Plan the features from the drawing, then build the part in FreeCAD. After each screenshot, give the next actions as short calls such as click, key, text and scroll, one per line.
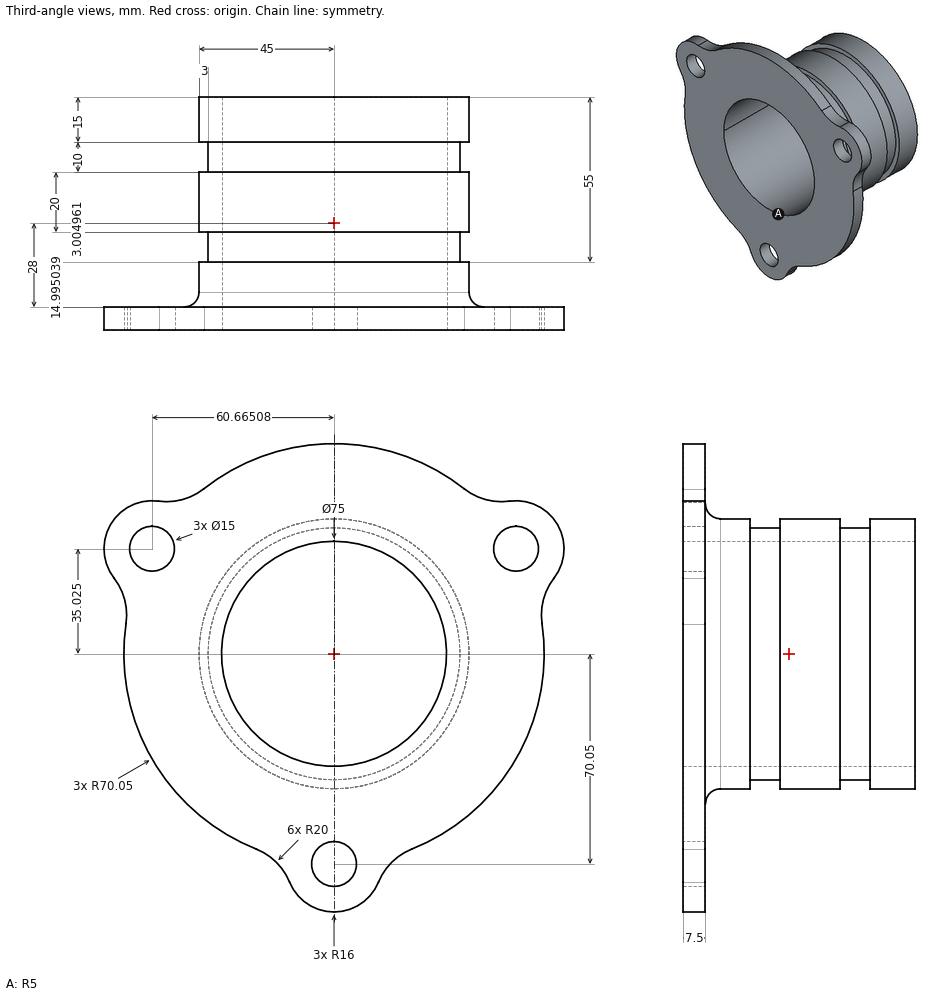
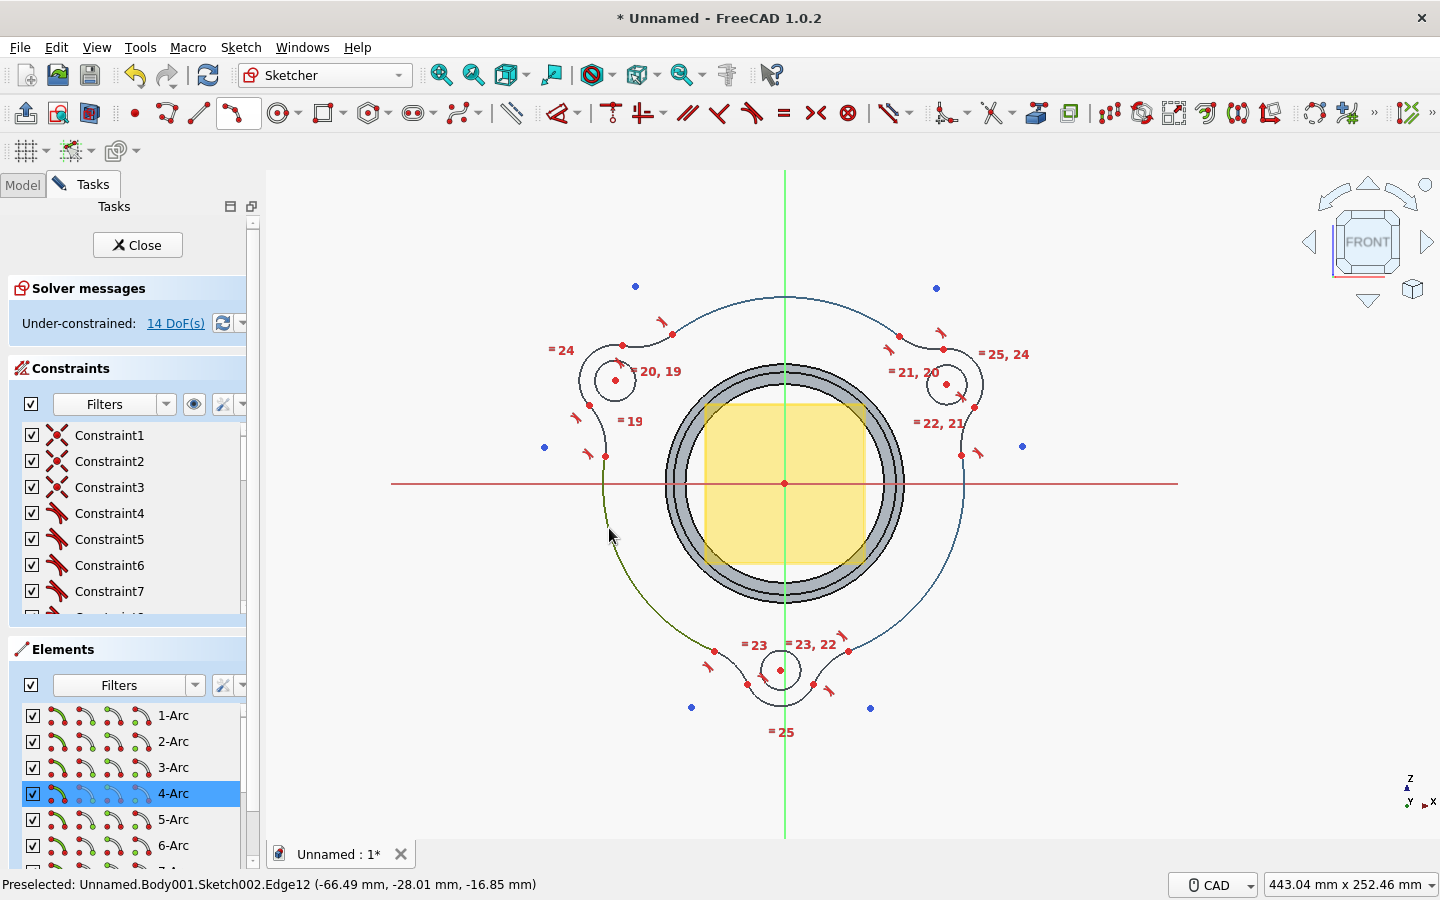
click(784, 114)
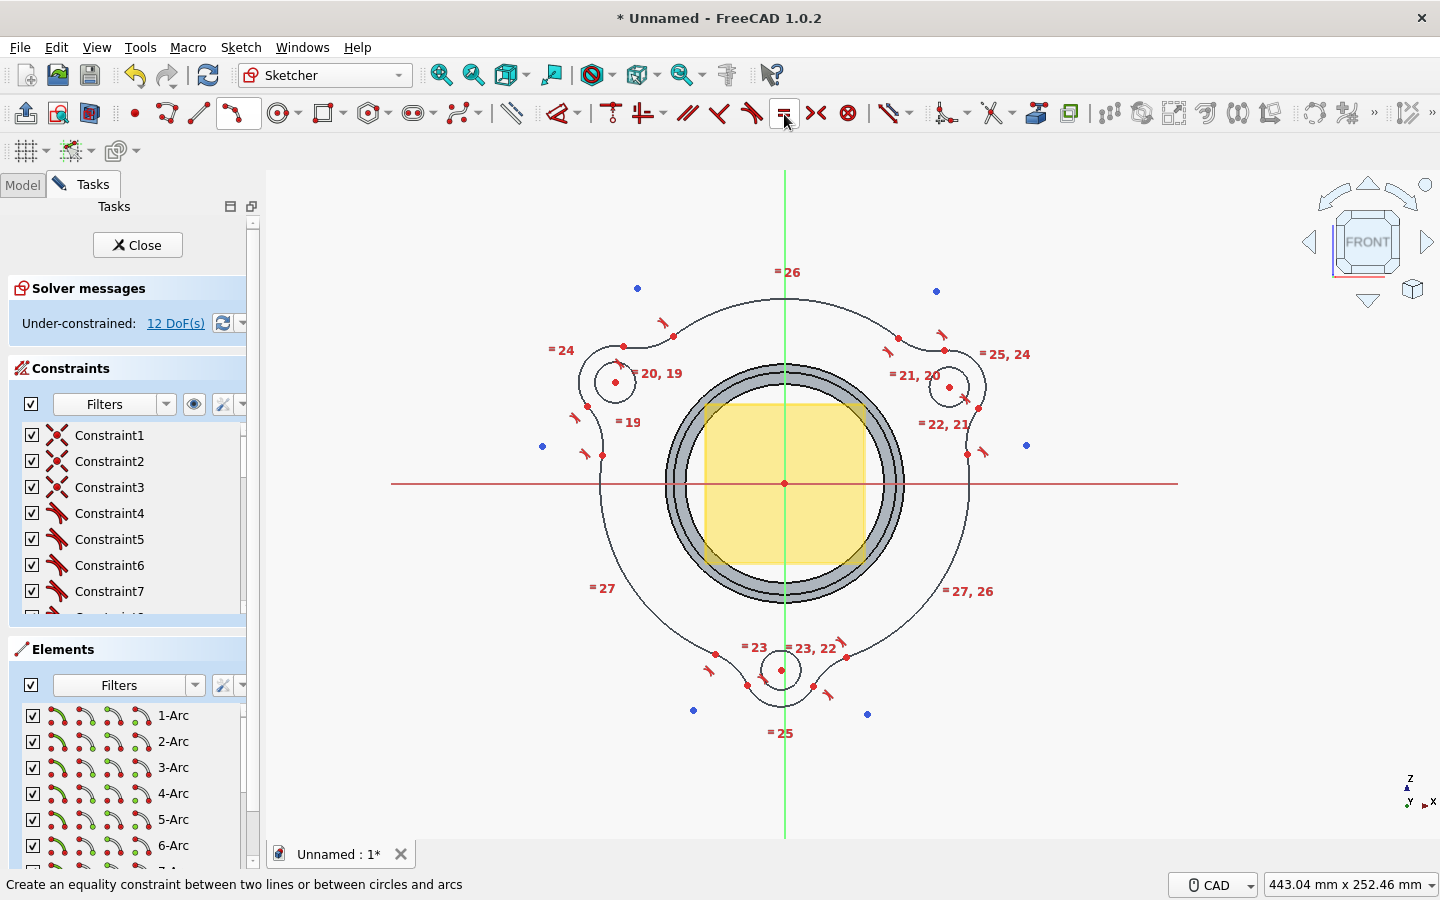
click(601, 368)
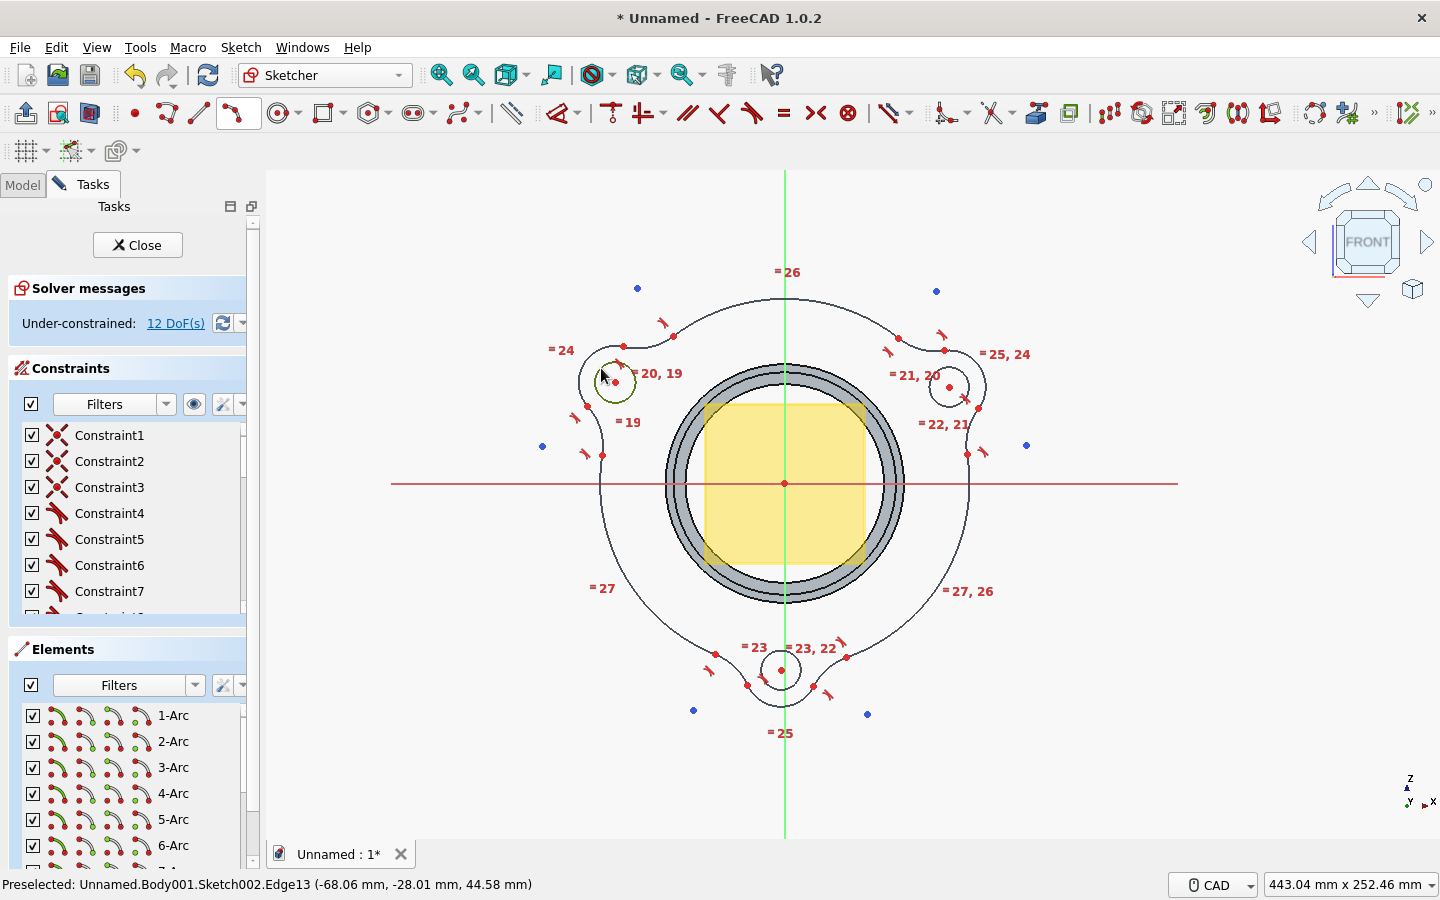
click(963, 373)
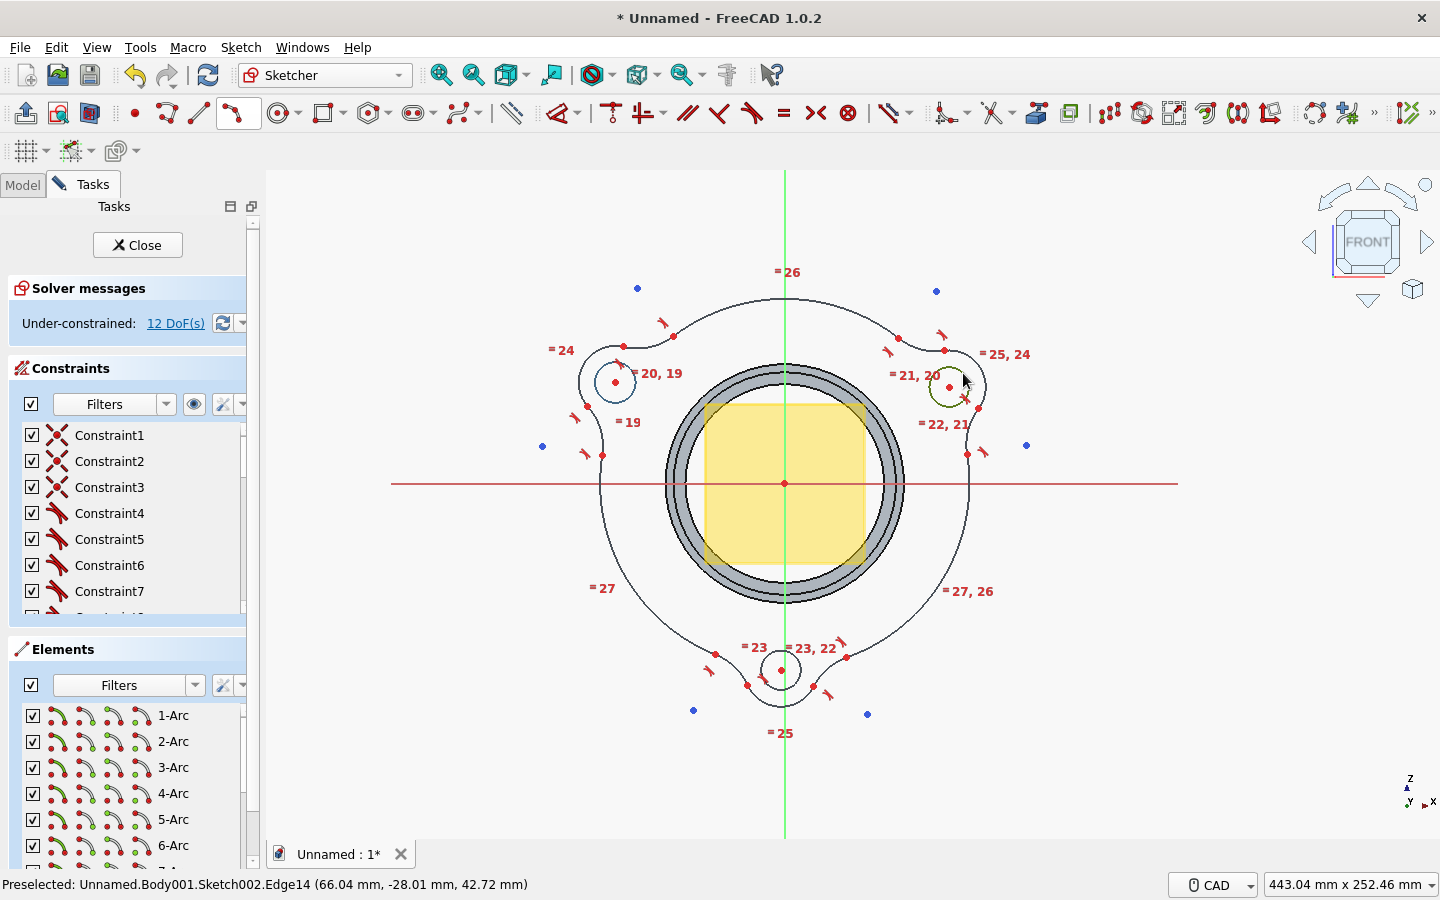
scroll(795, 656, up, 2)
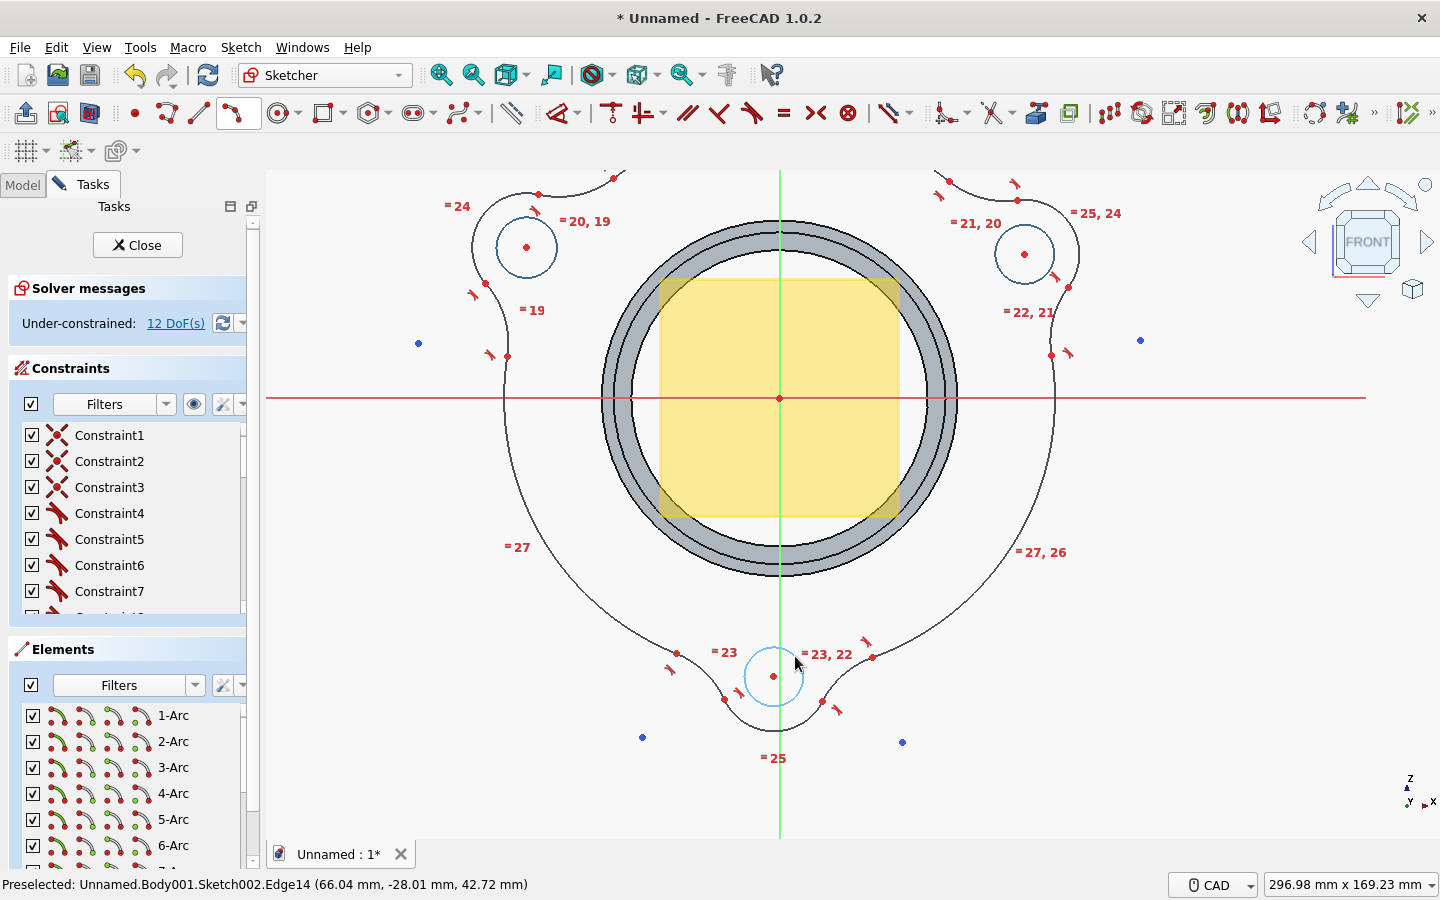
click(795, 656)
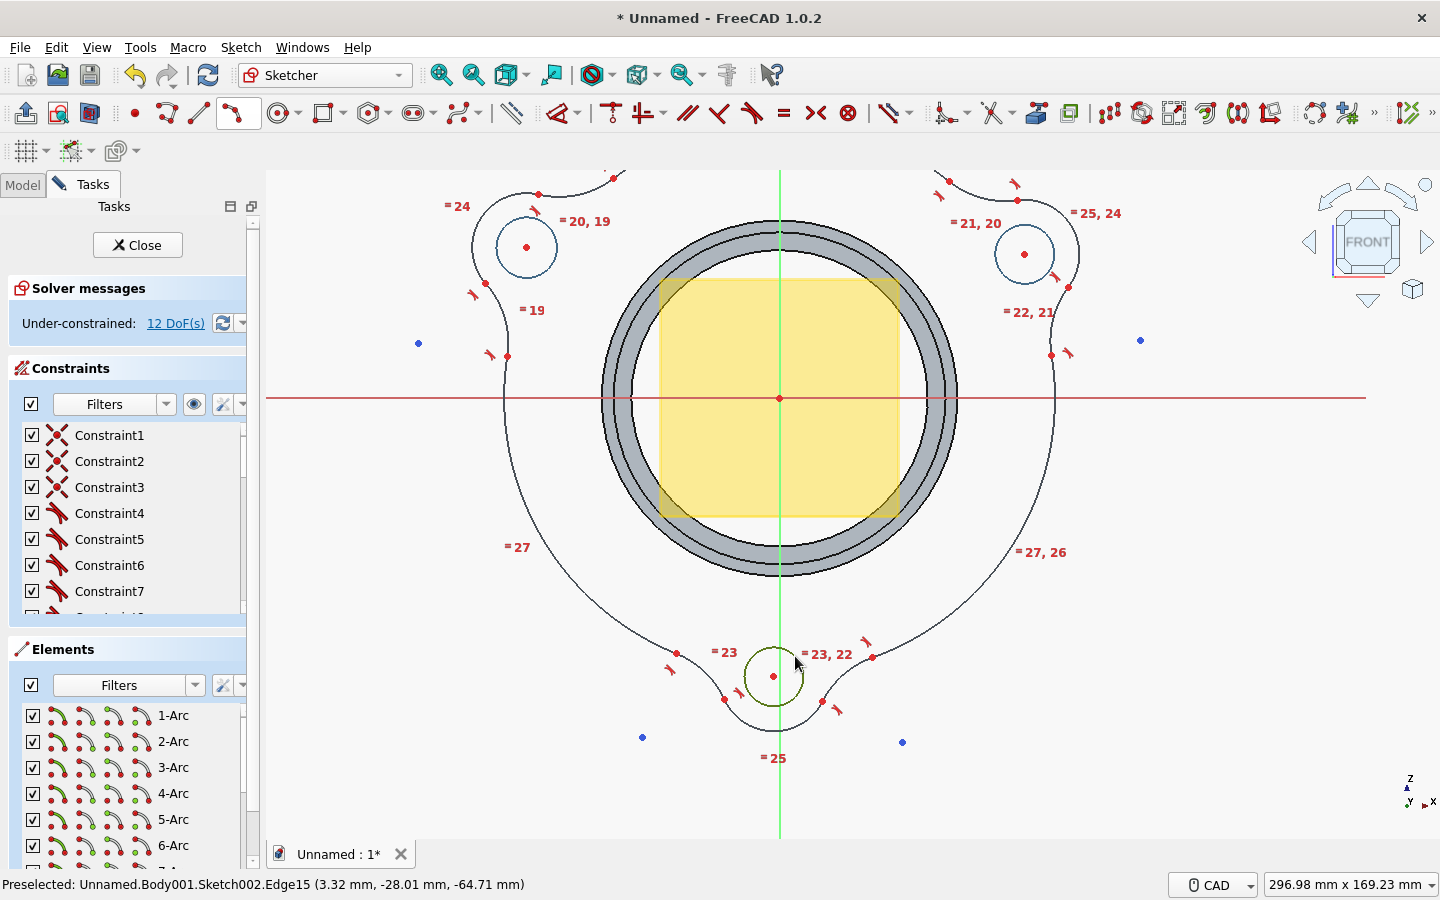
click(784, 114)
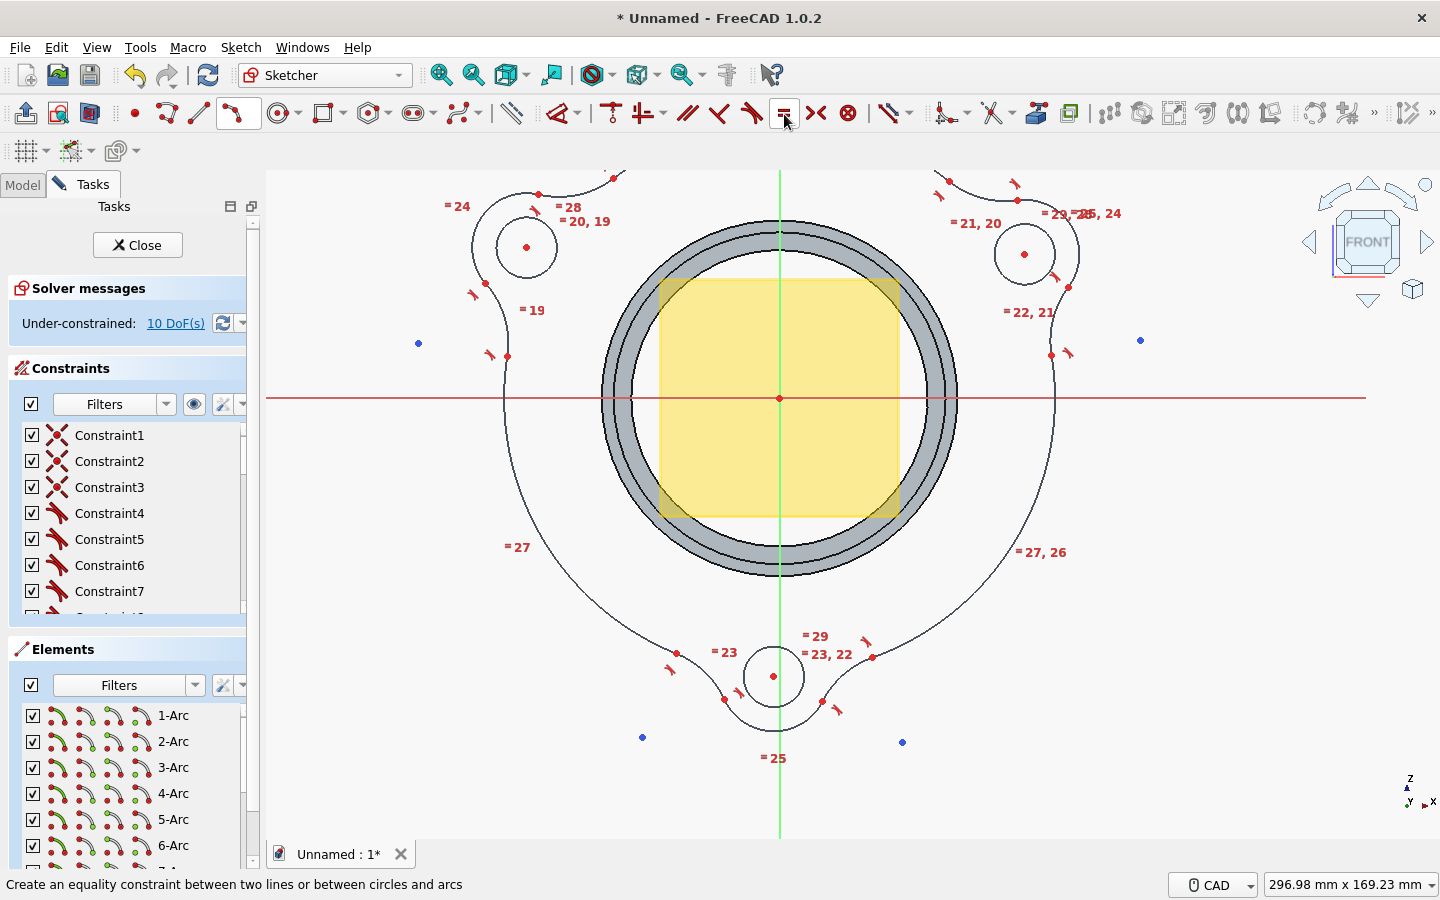
click(774, 677)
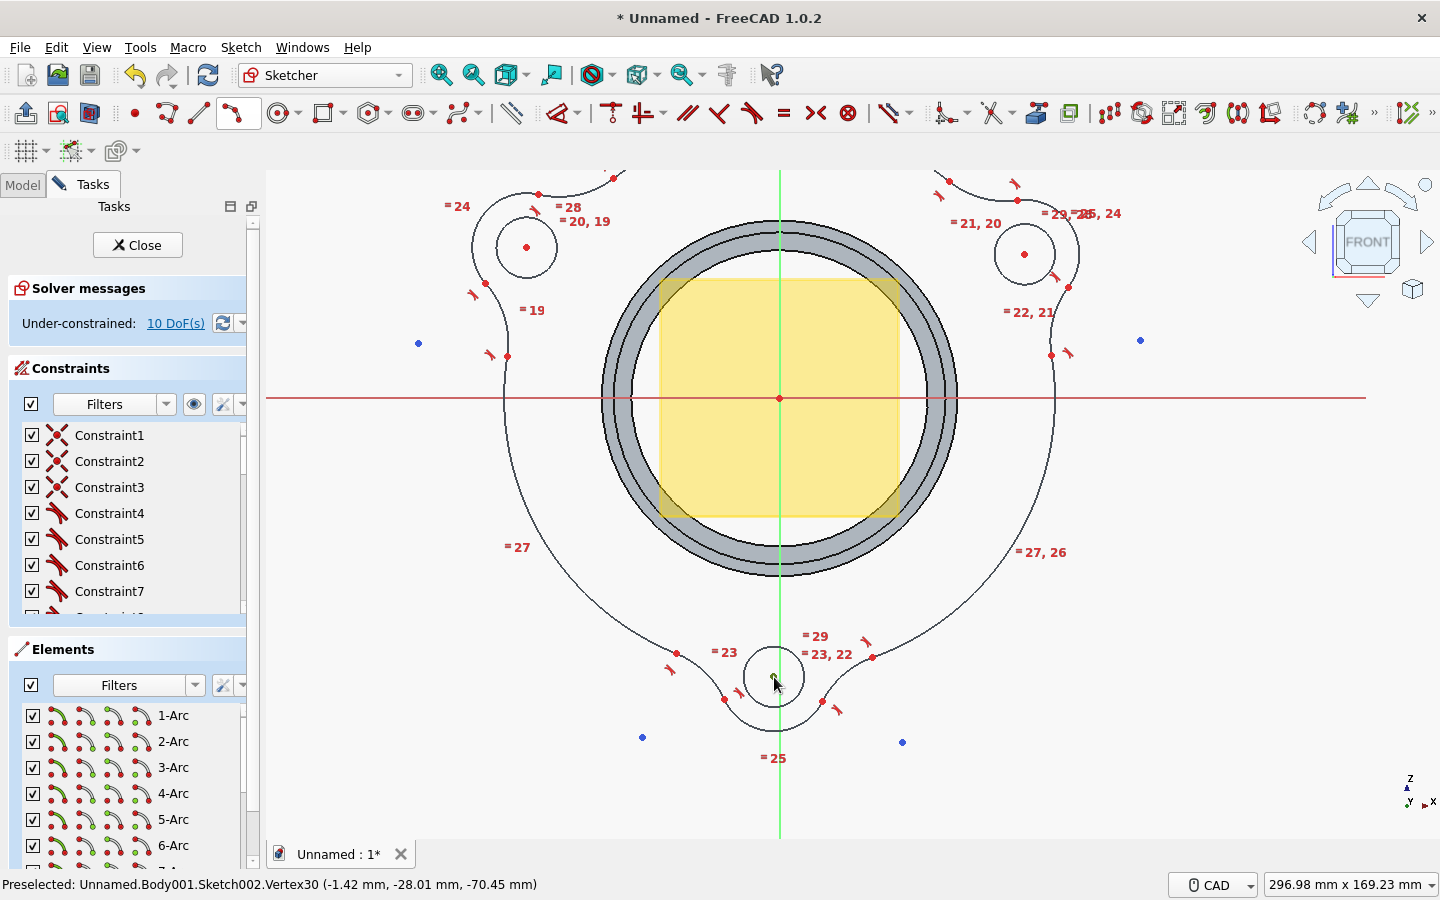
click(780, 767)